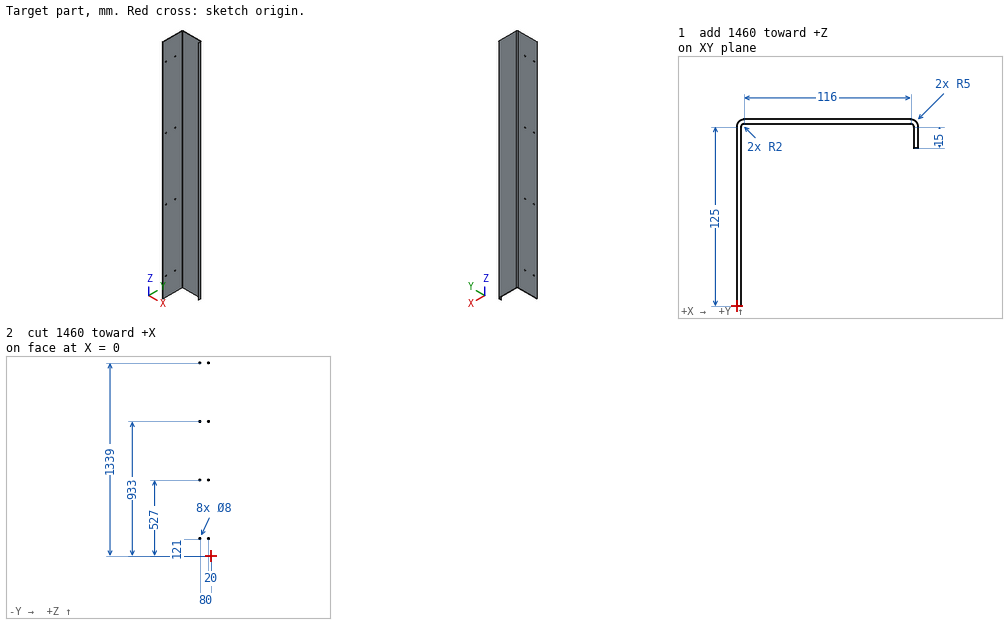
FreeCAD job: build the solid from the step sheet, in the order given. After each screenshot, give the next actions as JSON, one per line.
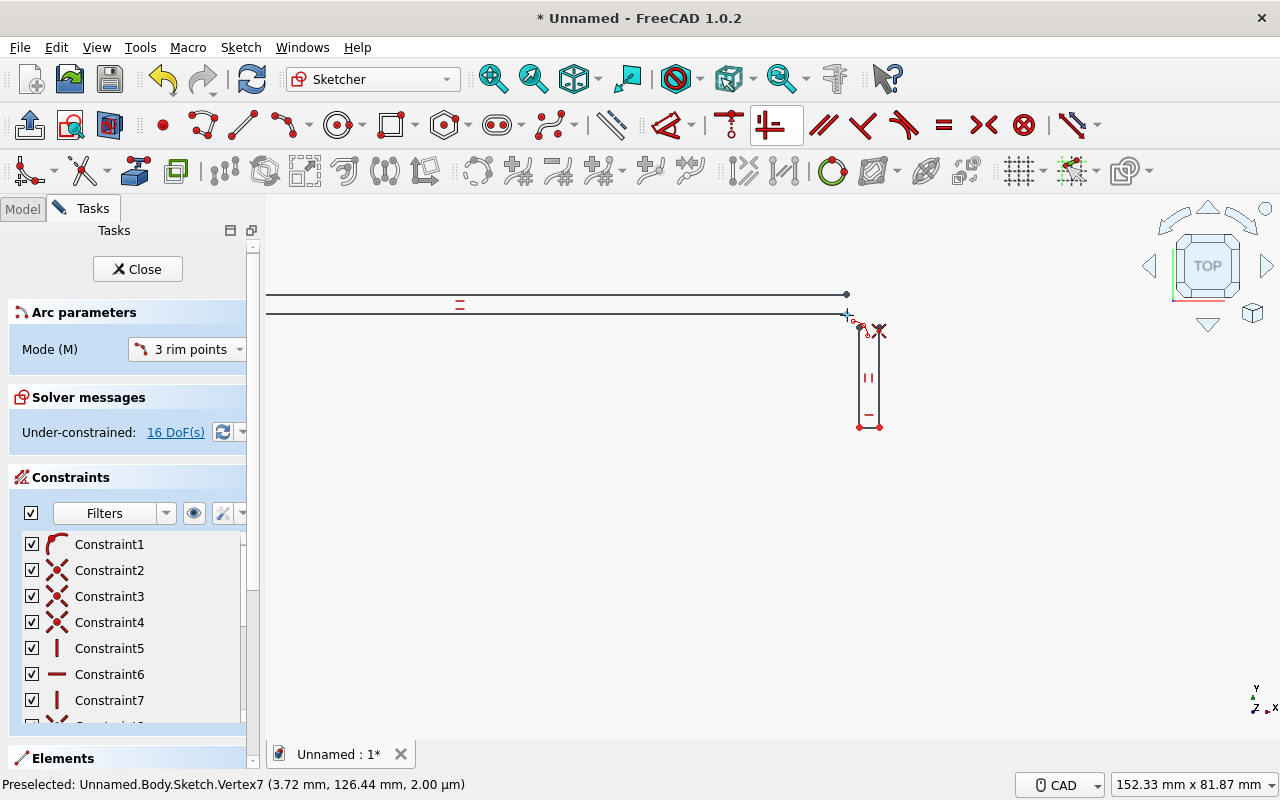
{"action": "left_click", "coordinate": [847, 314]}
{"action": "left_click", "coordinate": [859, 328]}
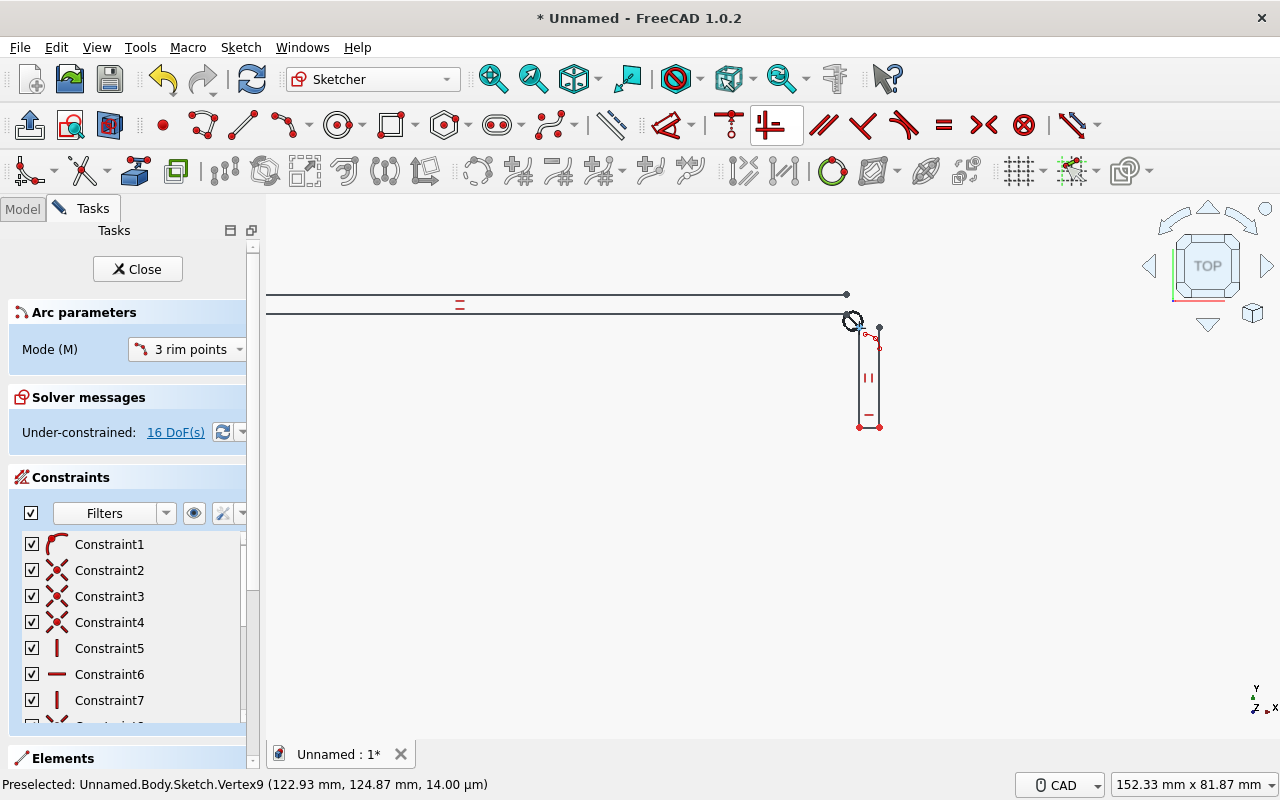
{"action": "scroll", "coordinate": [856, 318], "scroll_direction": "up", "scroll_amount": 8}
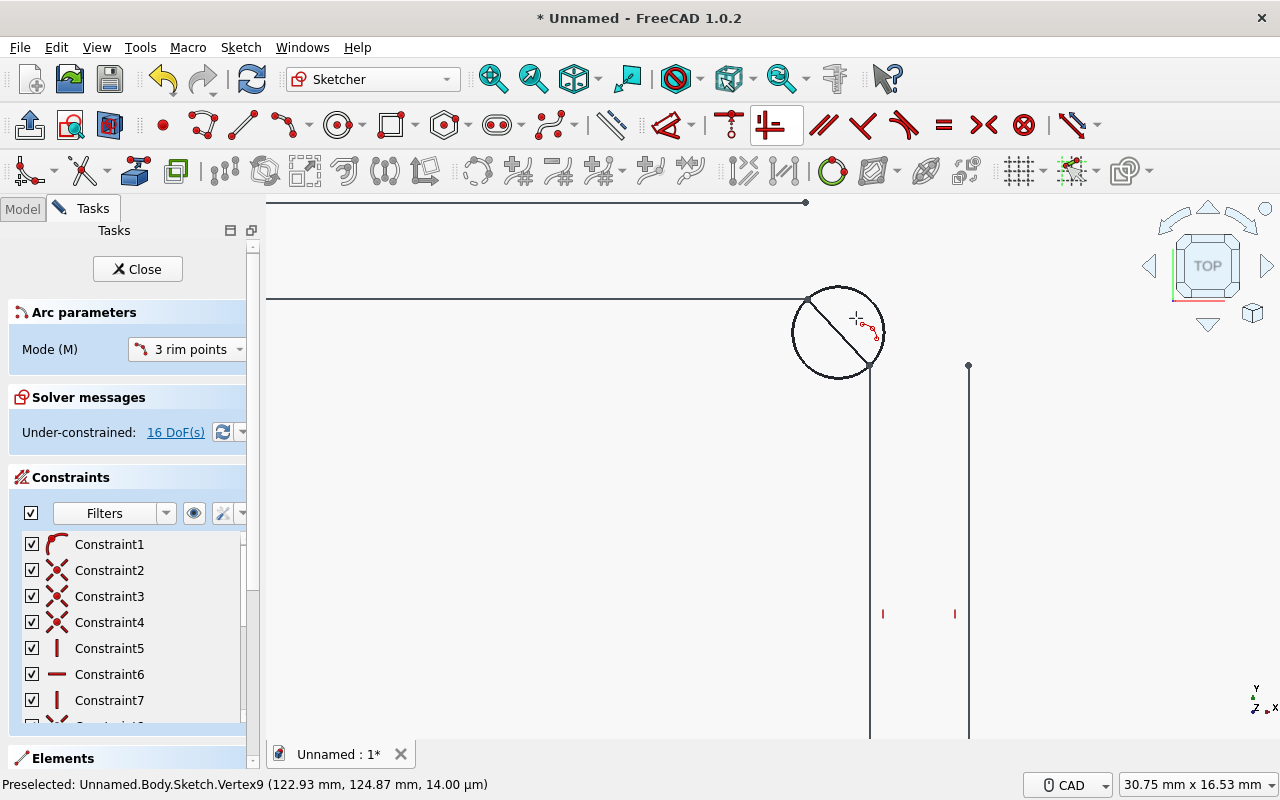
{"action": "left_click", "coordinate": [852, 315]}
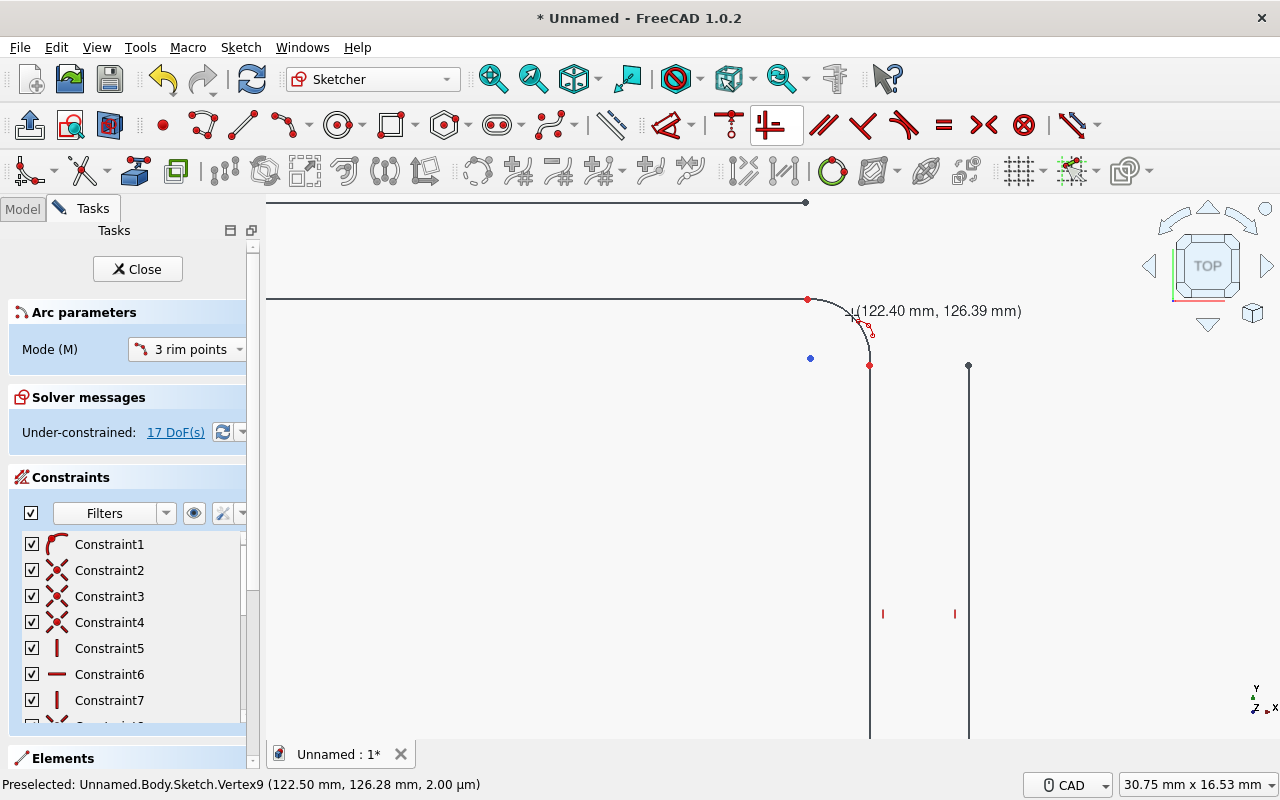
{"action": "scroll", "coordinate": [850, 316], "scroll_direction": "down", "scroll_amount": 13}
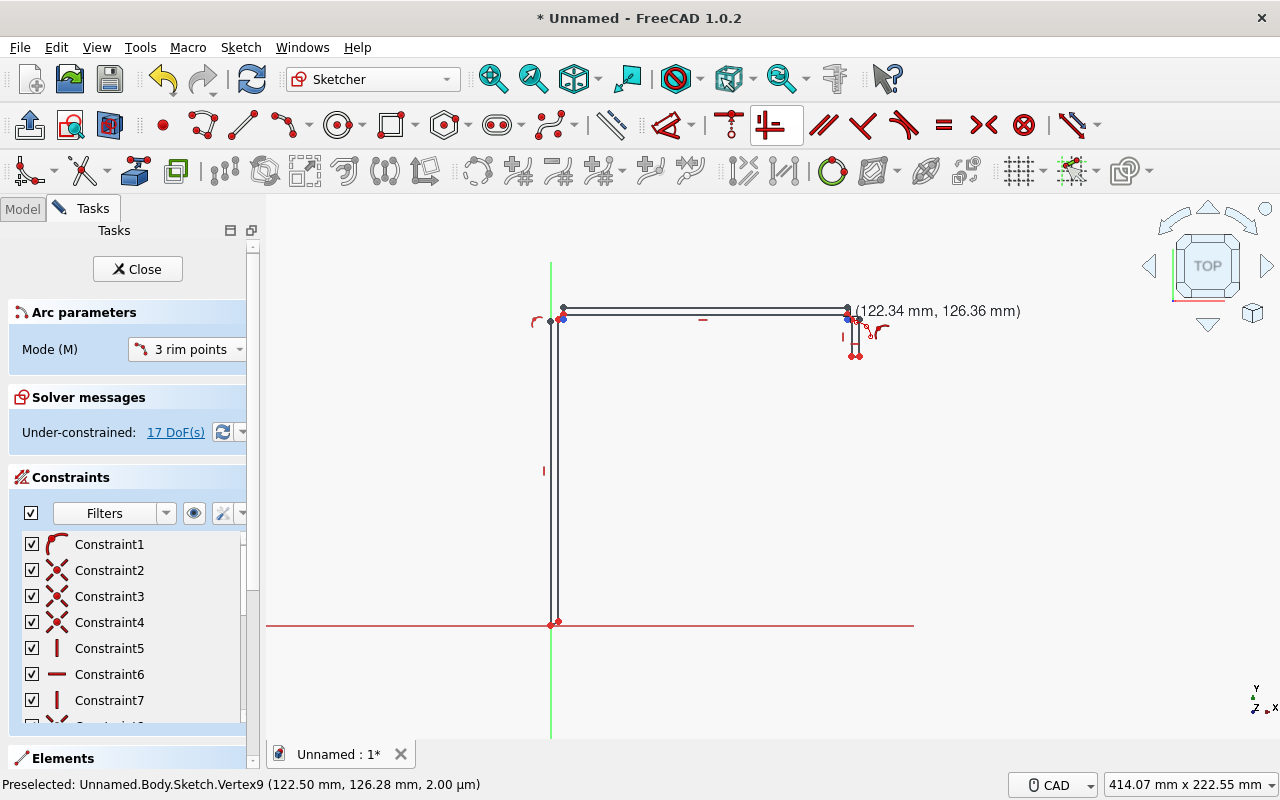
{"action": "scroll", "coordinate": [859, 320], "scroll_direction": "up", "scroll_amount": 4}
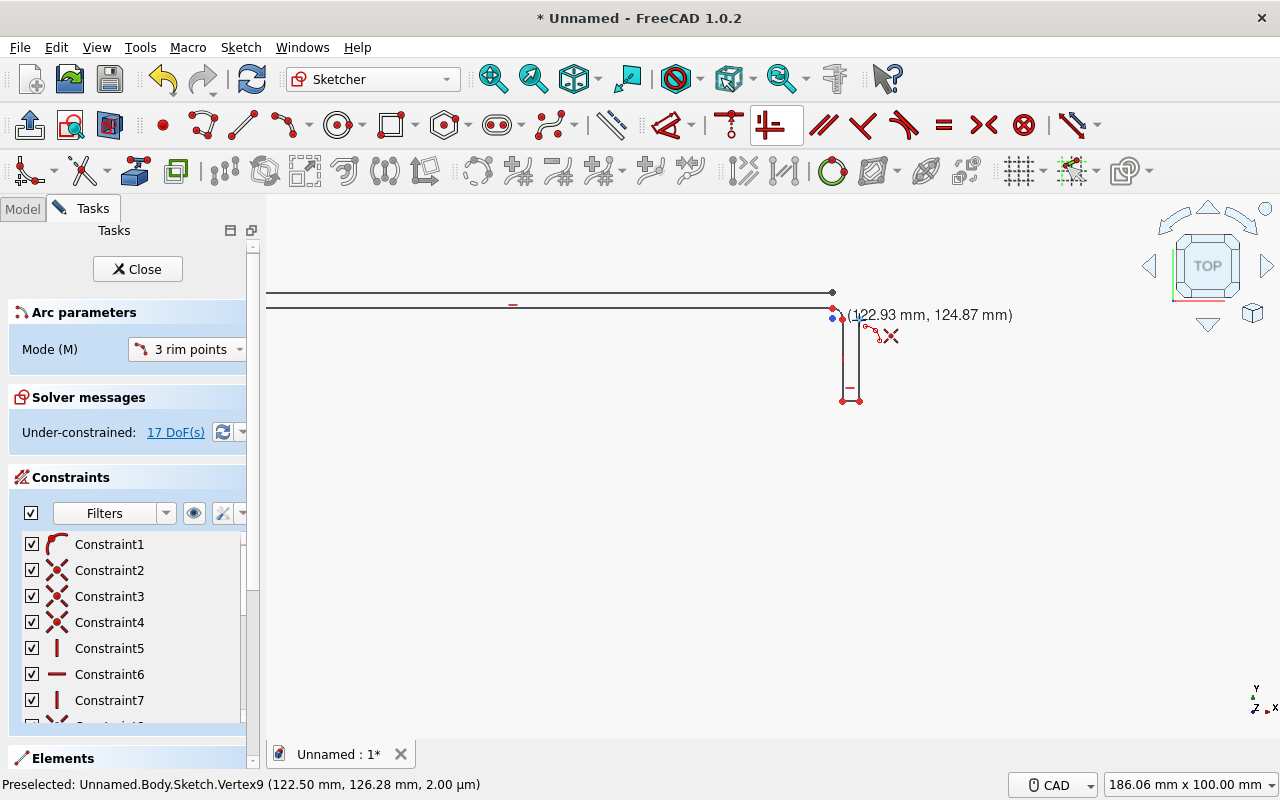
{"action": "left_click", "coordinate": [859, 320]}
{"action": "left_click", "coordinate": [832, 293]}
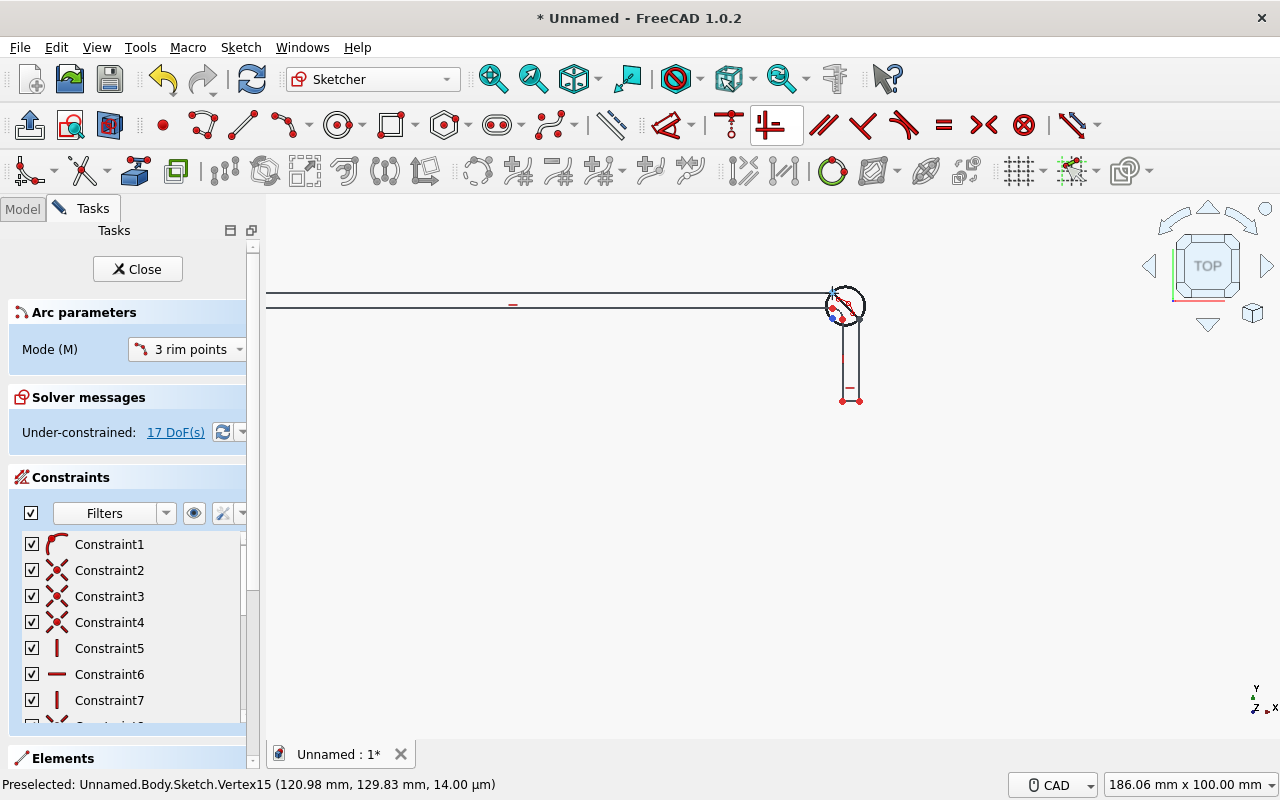
{"action": "scroll", "coordinate": [851, 300], "scroll_direction": "up", "scroll_amount": 4}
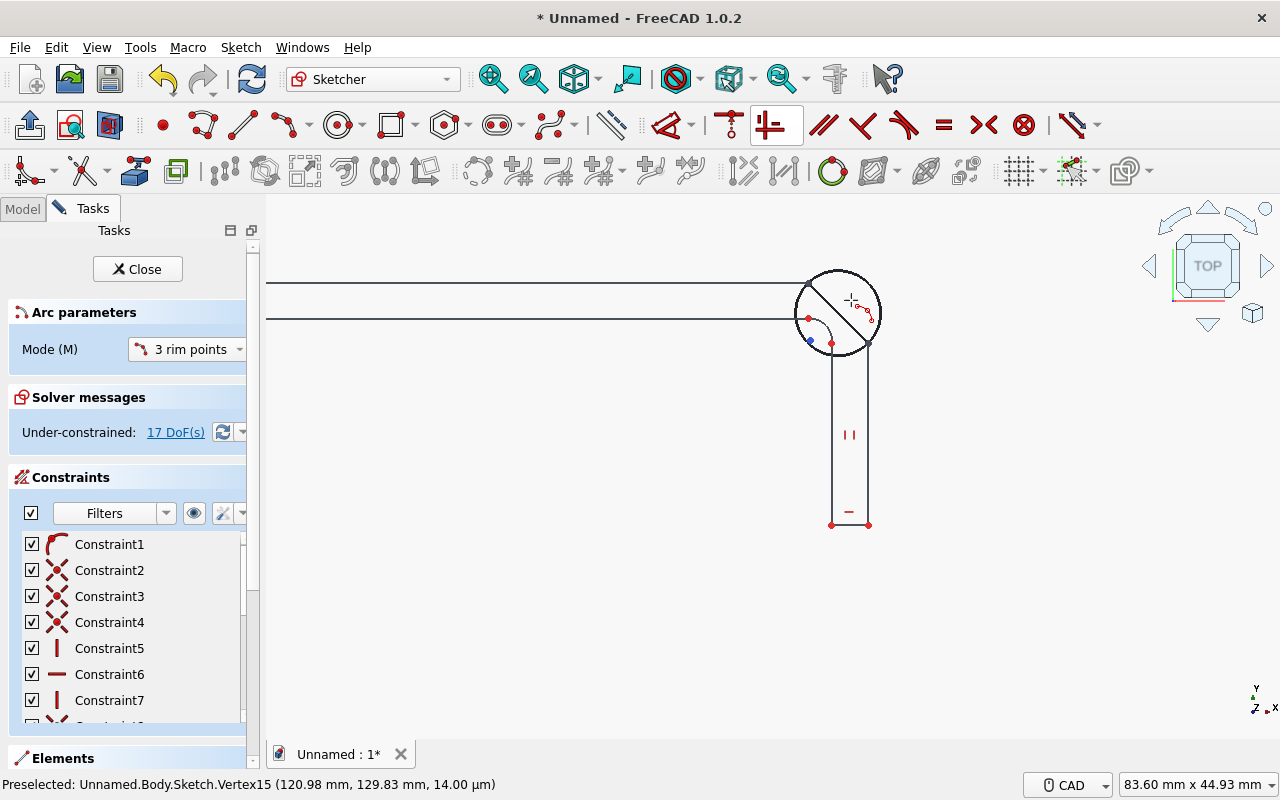
{"action": "left_click", "coordinate": [851, 299]}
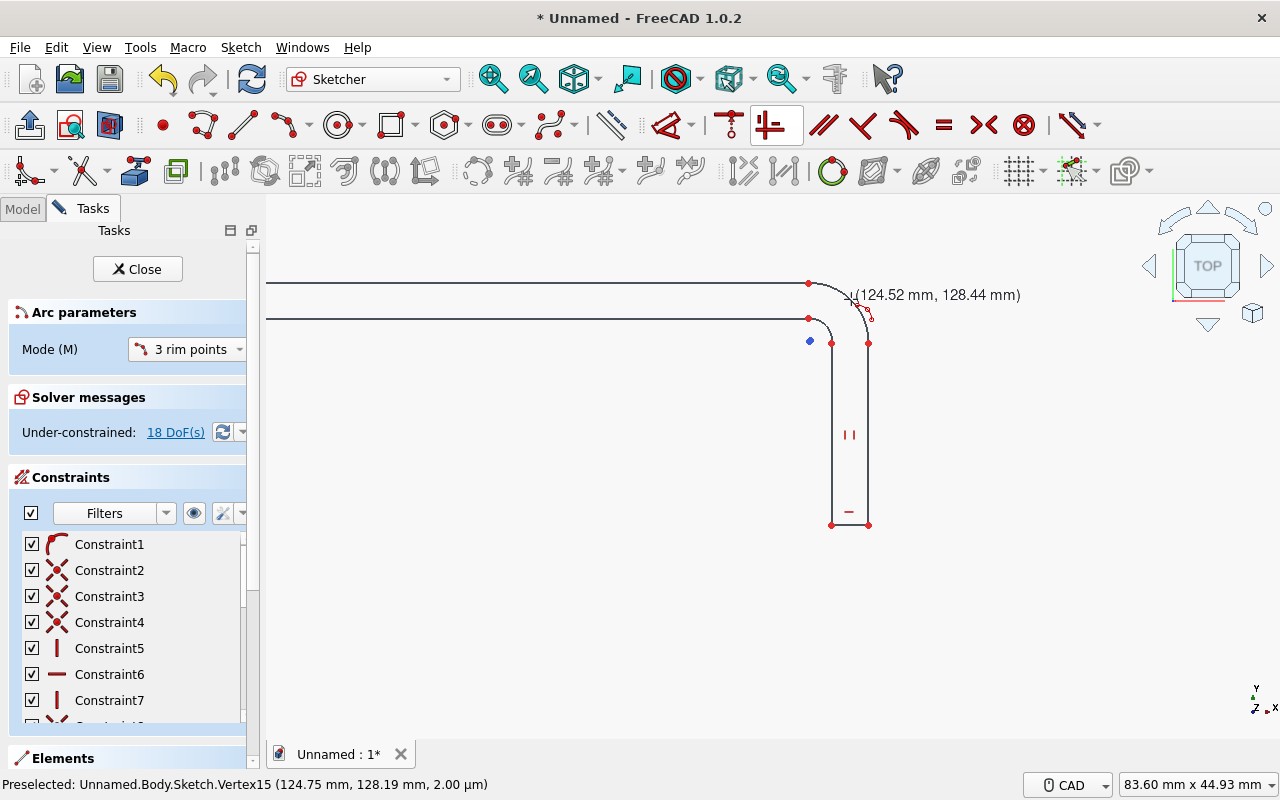
{"action": "scroll", "coordinate": [856, 314], "scroll_direction": "down", "scroll_amount": 8}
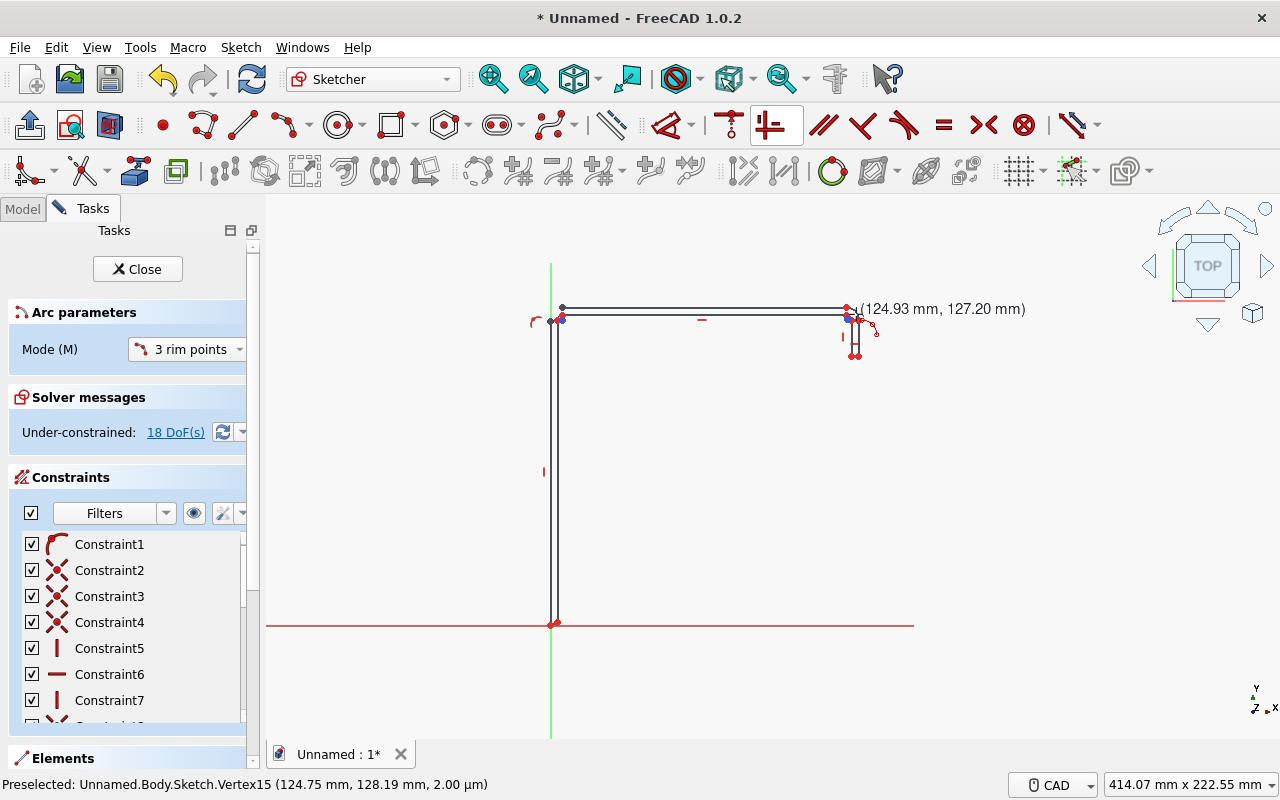
{"action": "scroll", "coordinate": [563, 308], "scroll_direction": "up", "scroll_amount": 4}